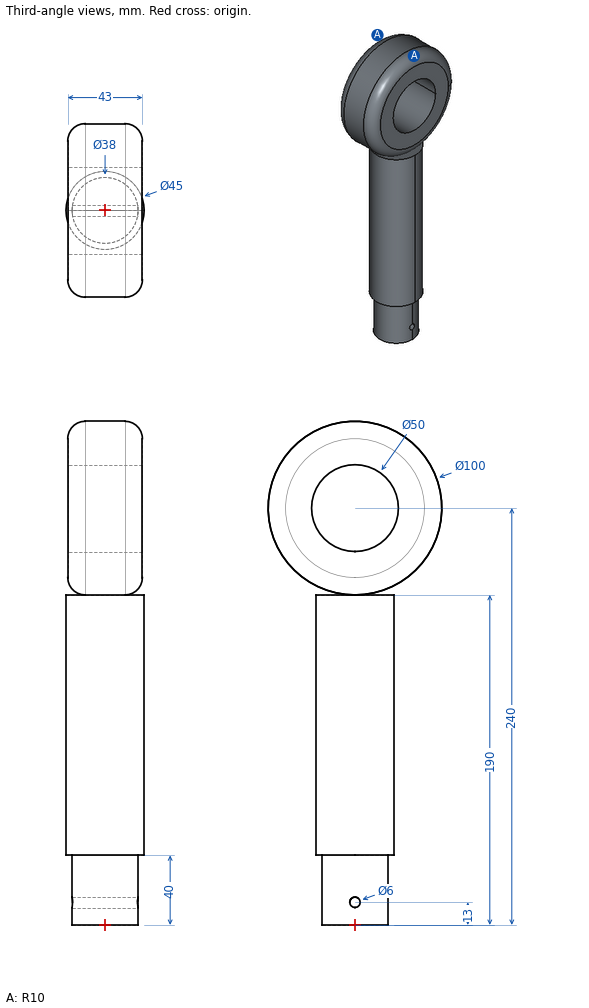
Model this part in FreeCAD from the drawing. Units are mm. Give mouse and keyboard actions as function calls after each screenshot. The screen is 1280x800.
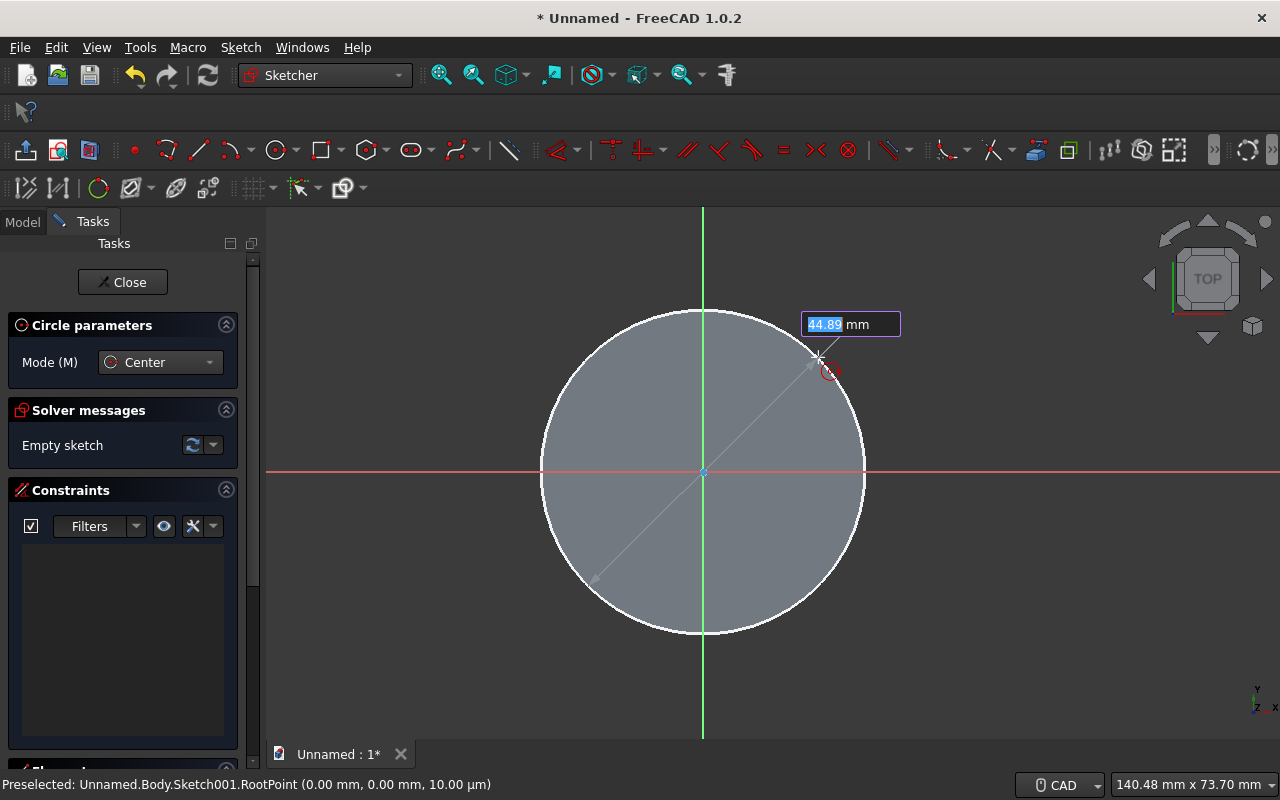
text(45)
key(Return)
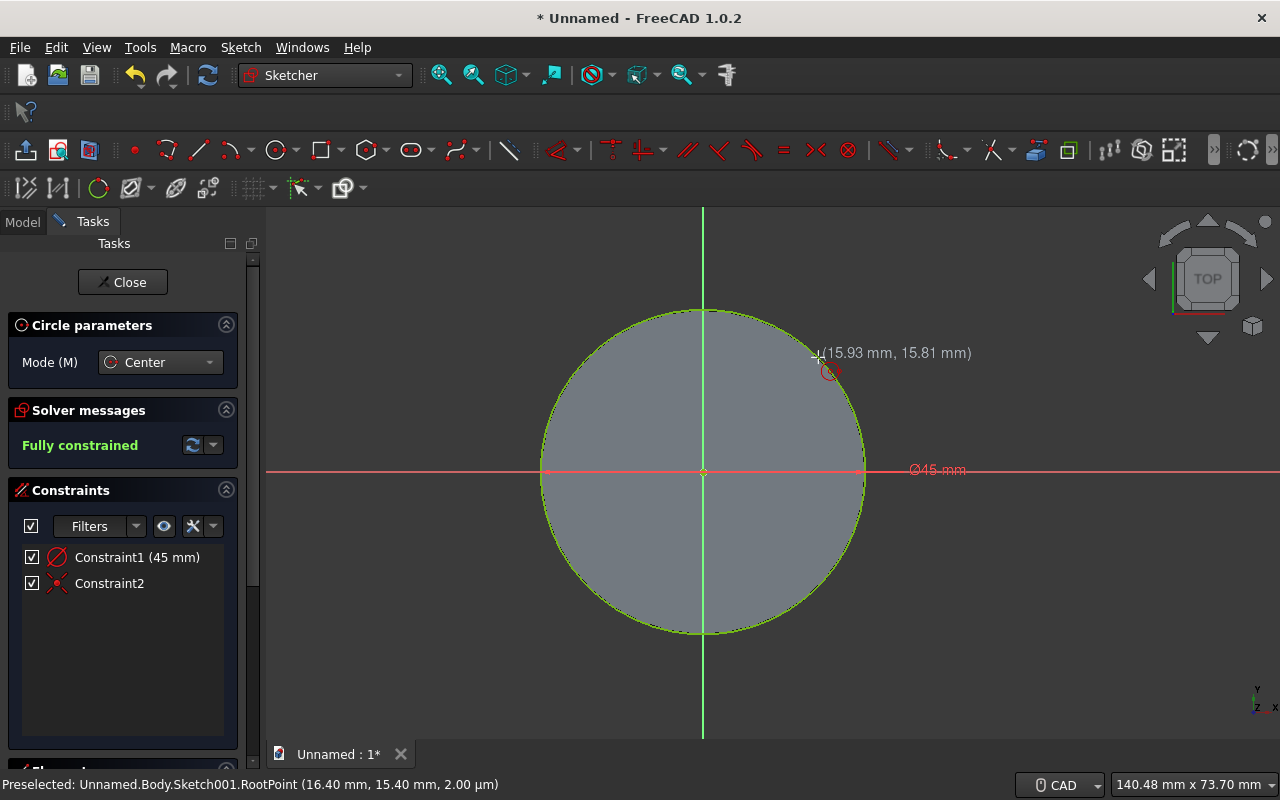
click(703, 472)
move(800, 375)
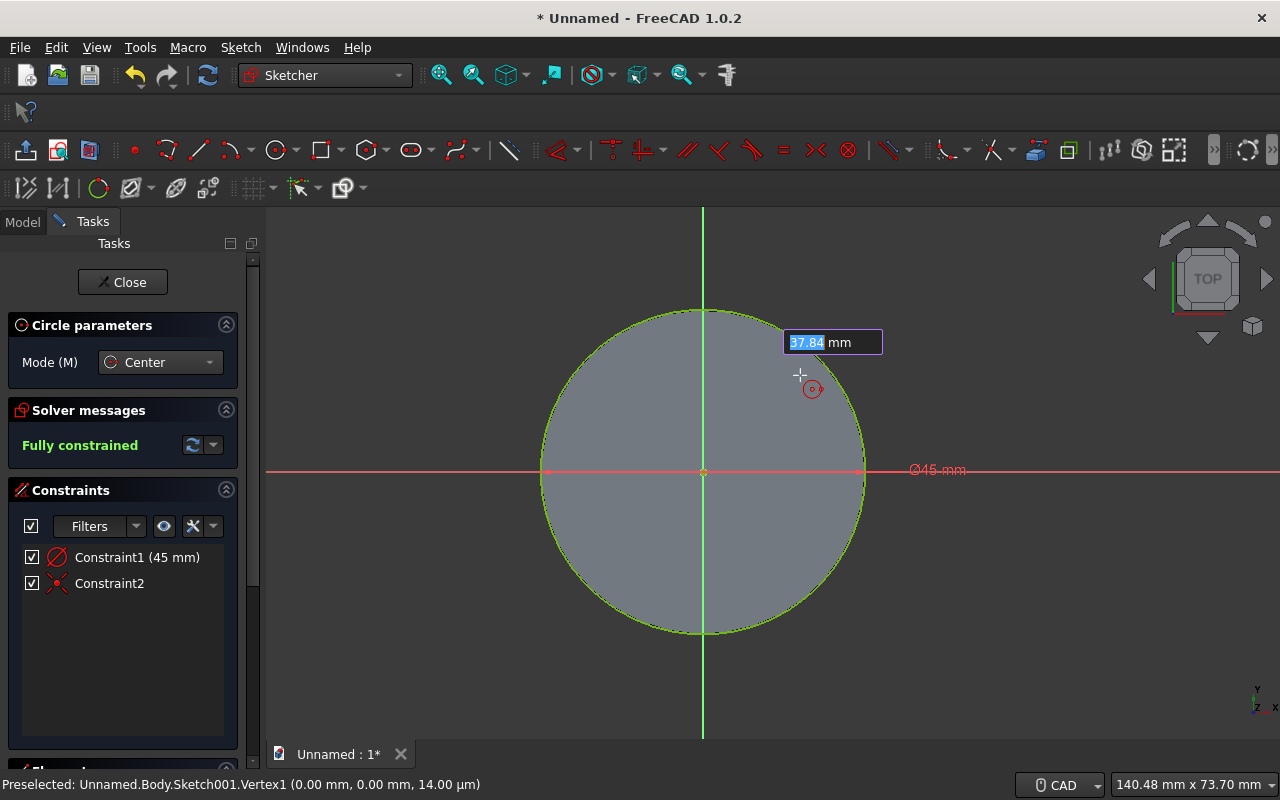
text(38)
key(Return)
key(Escape)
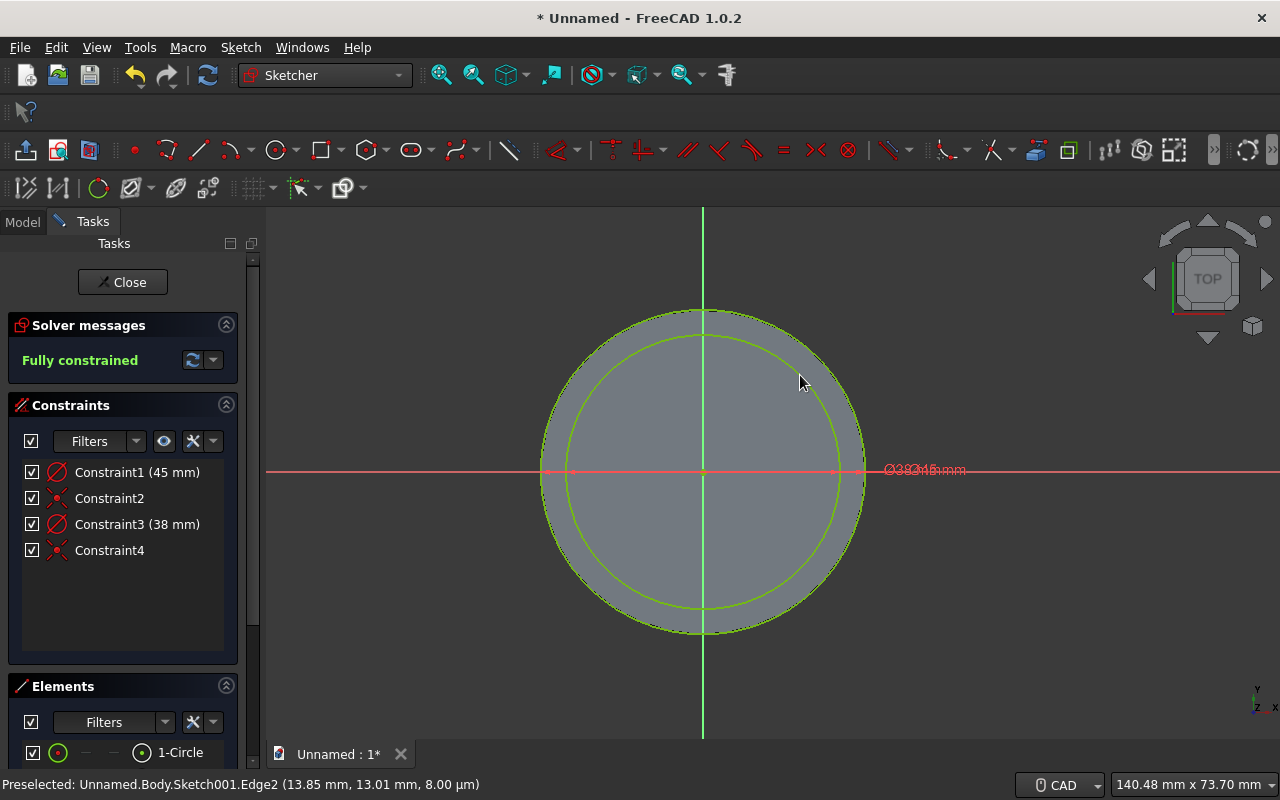
click(123, 282)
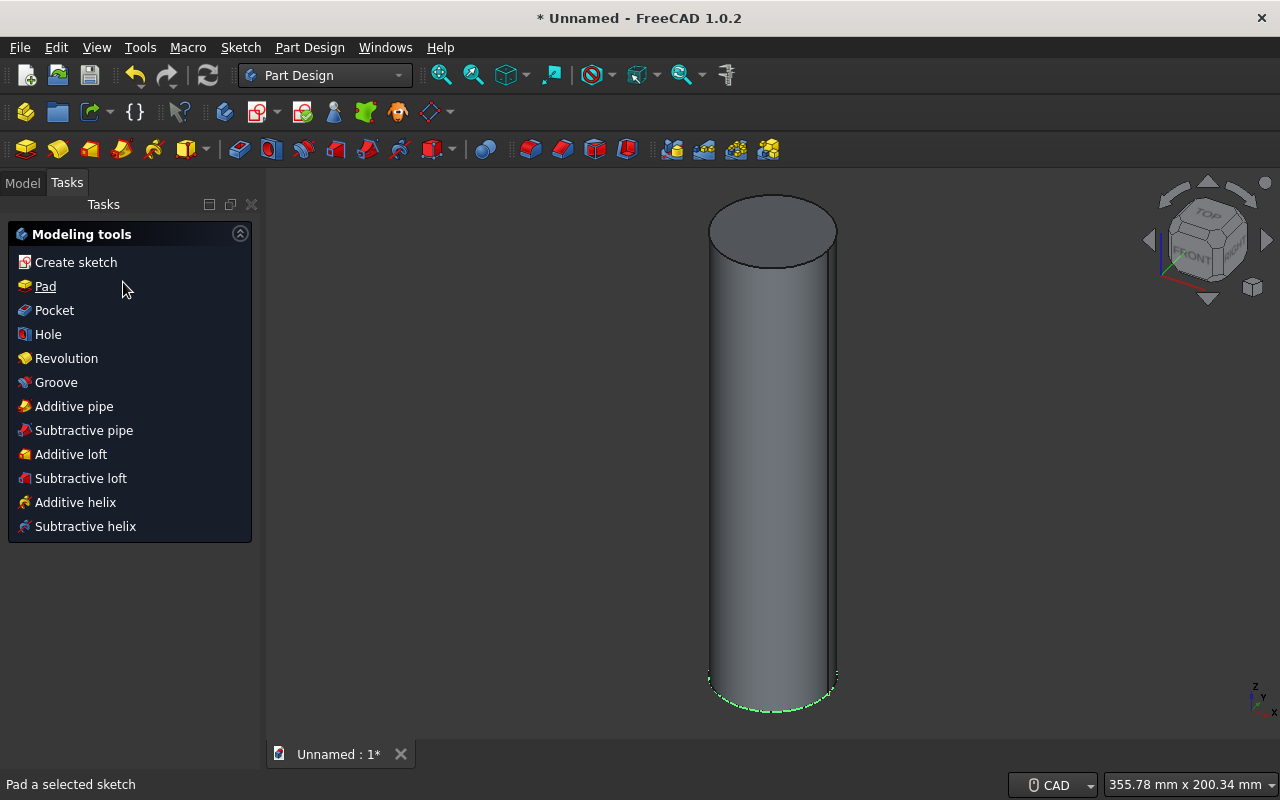
click(240, 150)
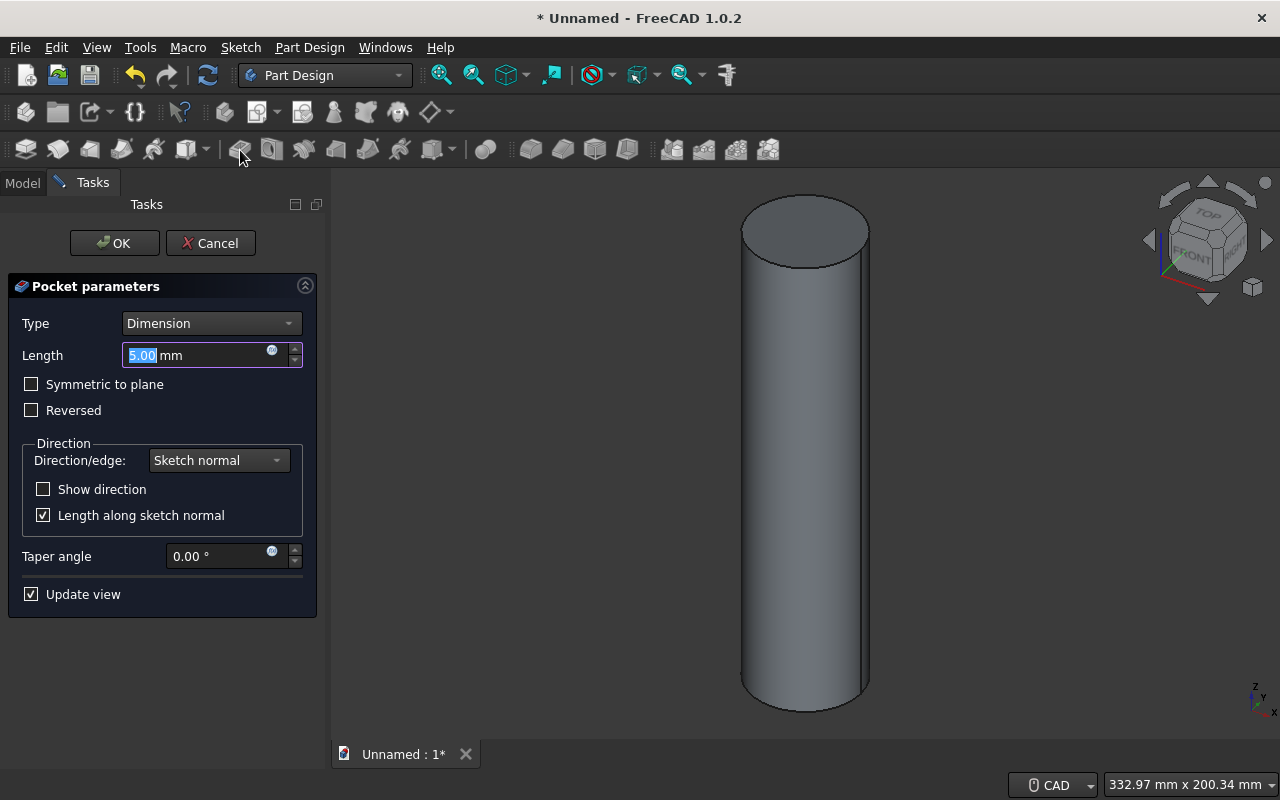
text(40)
key(Tab)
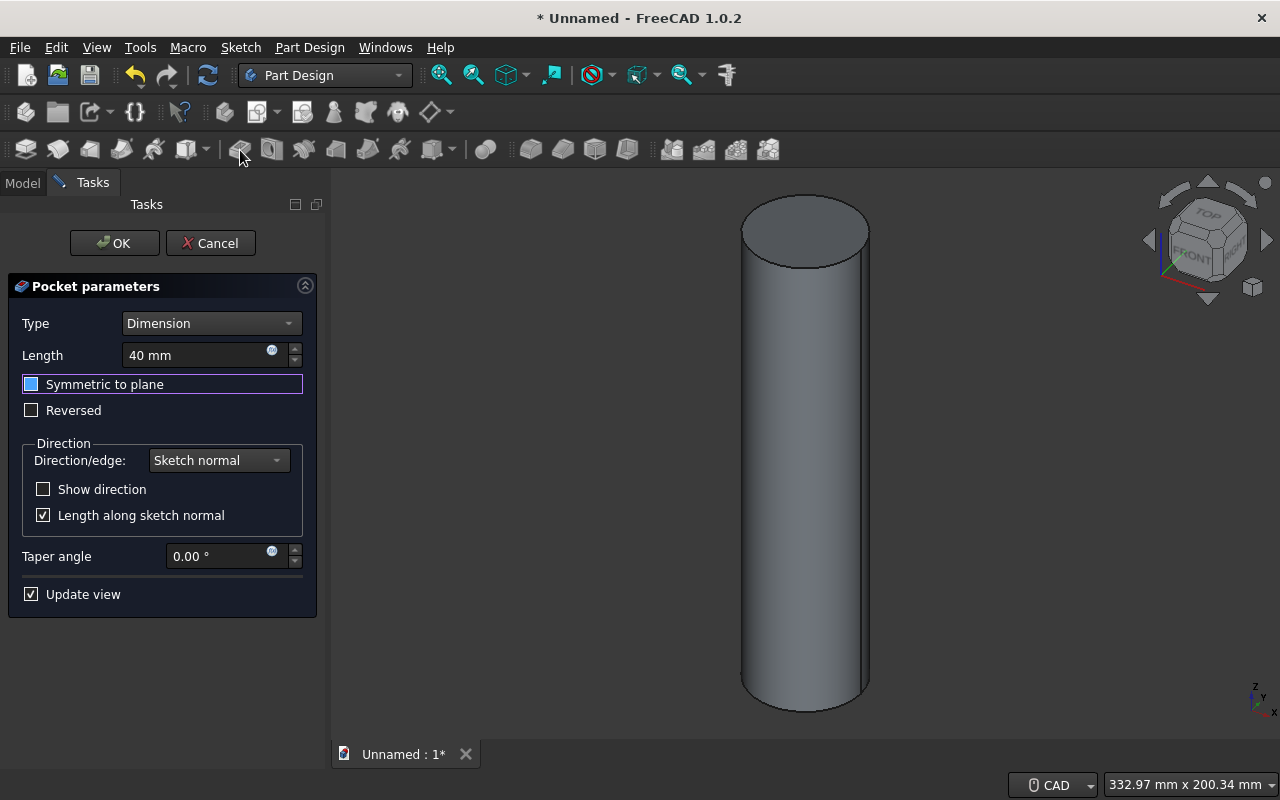
click(30, 410)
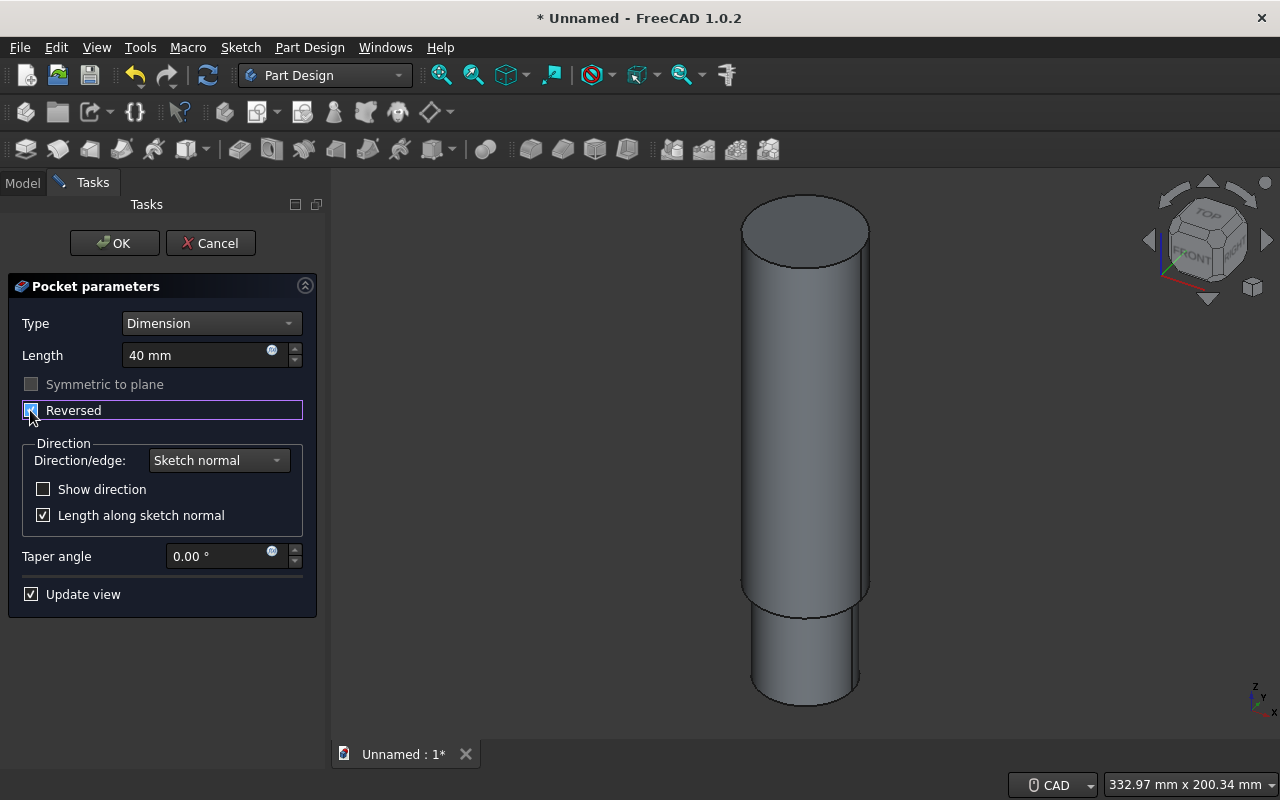
click(115, 243)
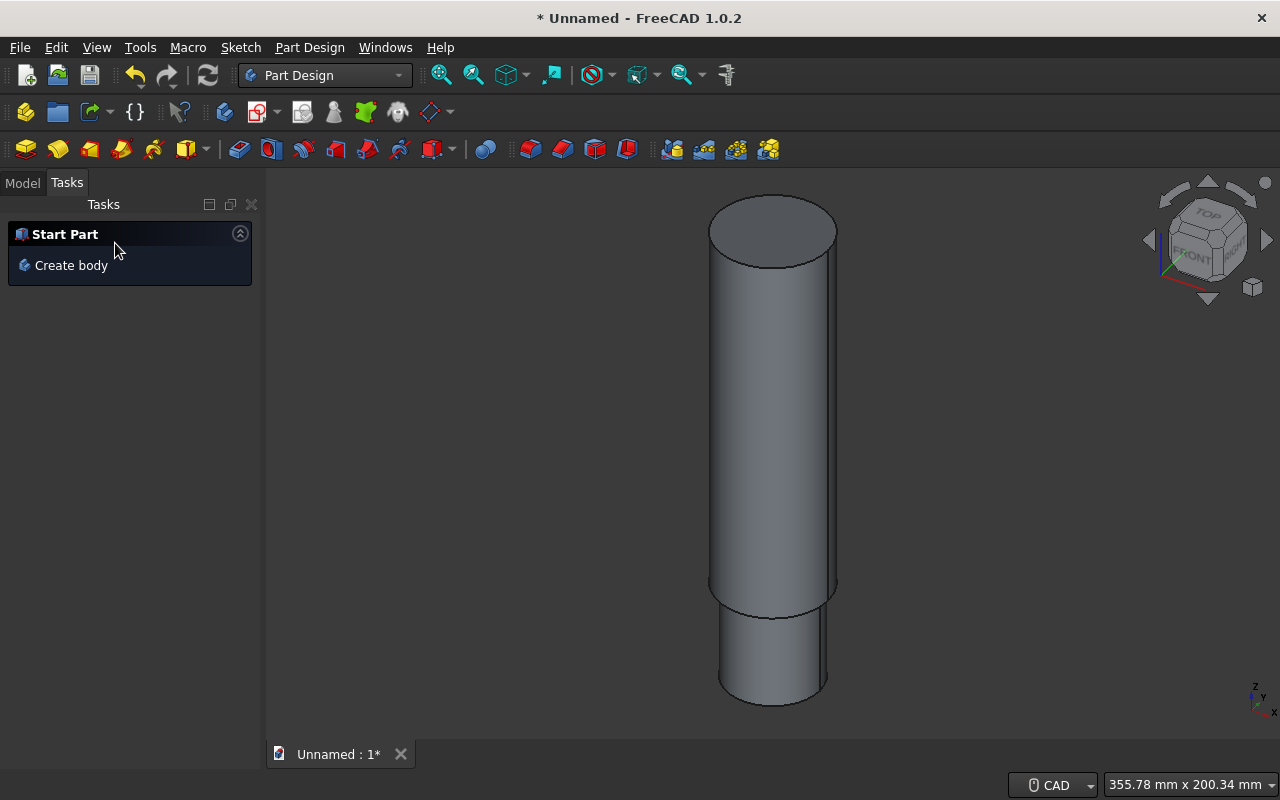
click(258, 112)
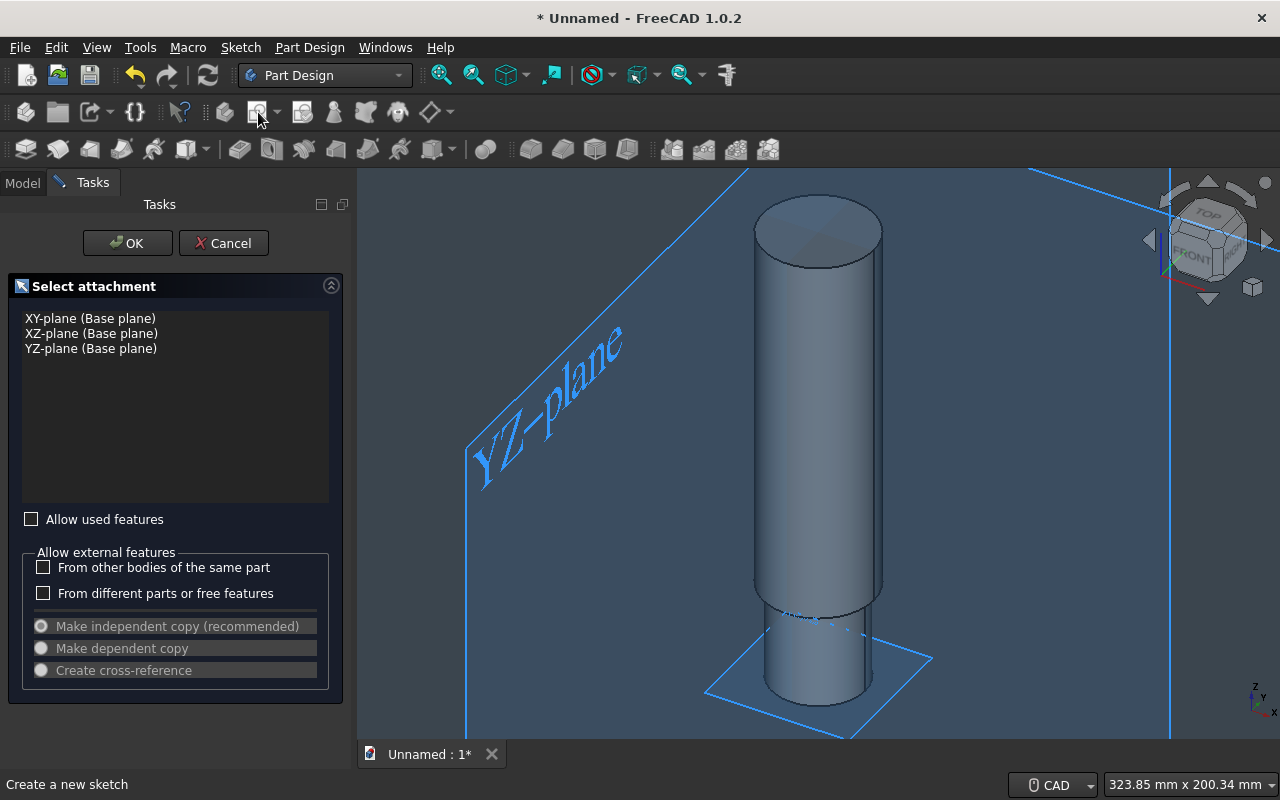
click(82, 348)